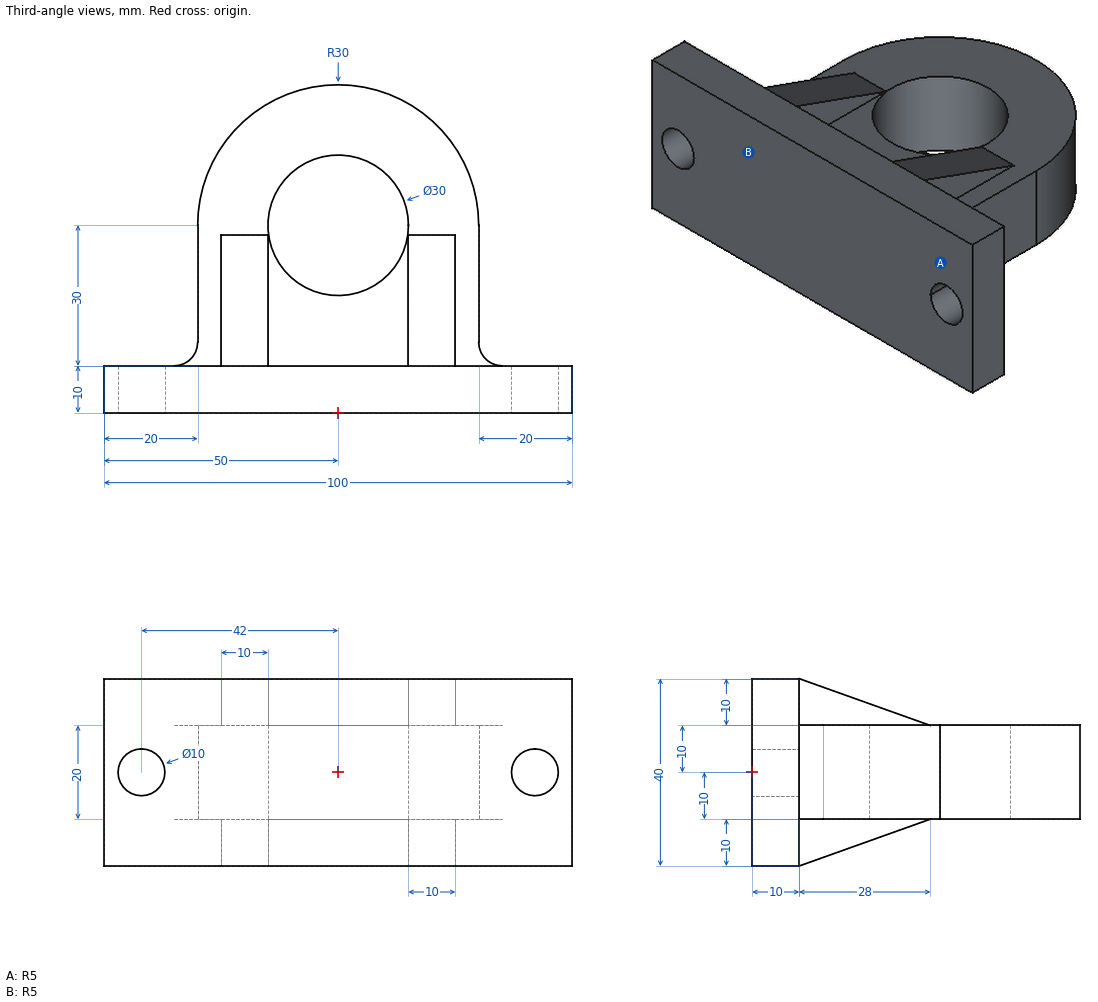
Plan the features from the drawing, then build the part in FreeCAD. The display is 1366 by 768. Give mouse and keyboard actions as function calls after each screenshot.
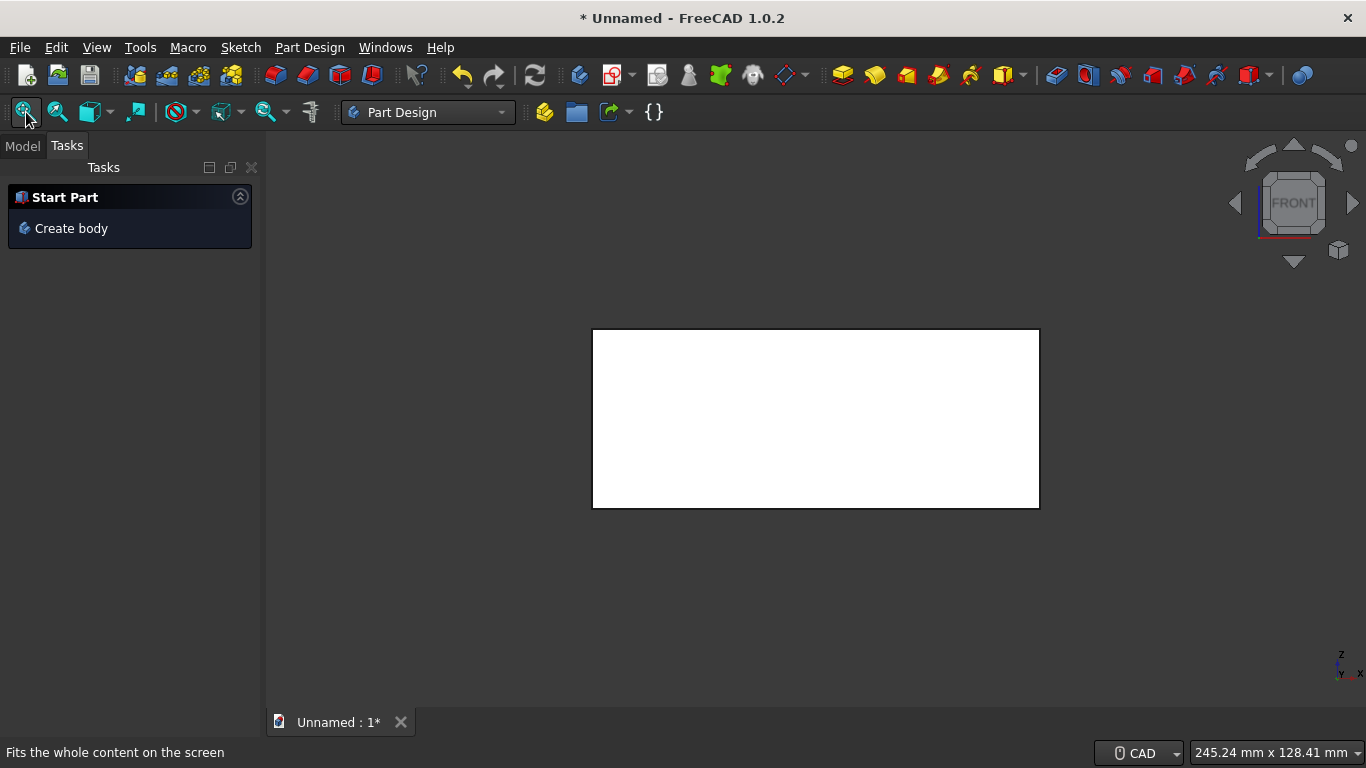
click(26, 112)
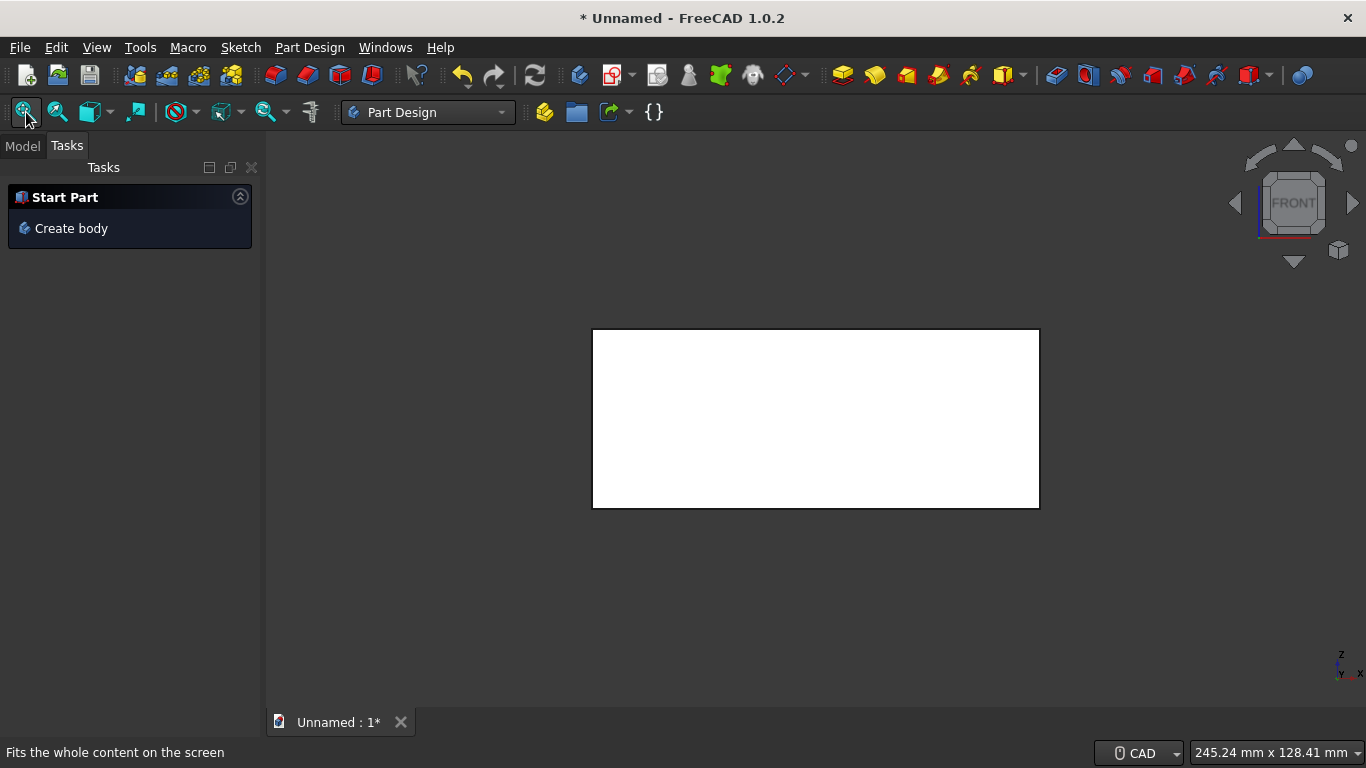
key(3)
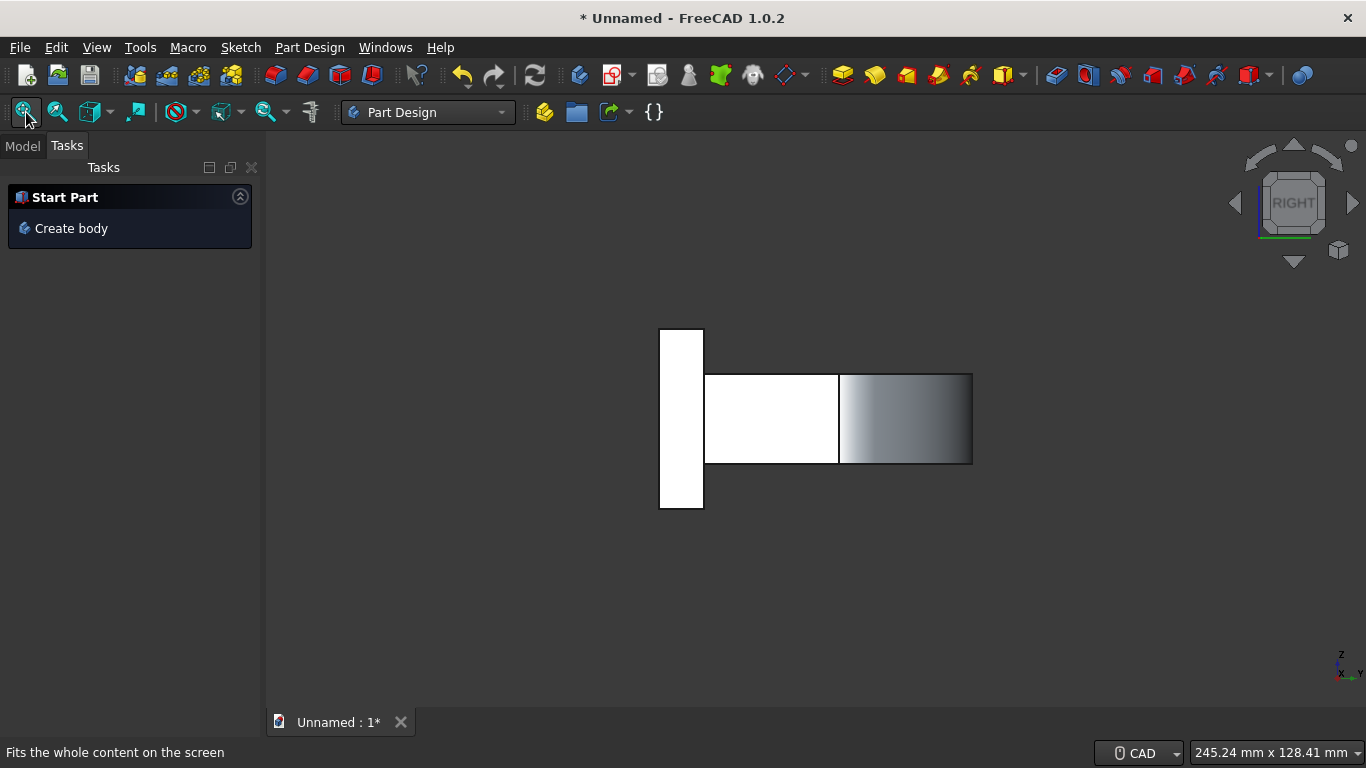
click(26, 112)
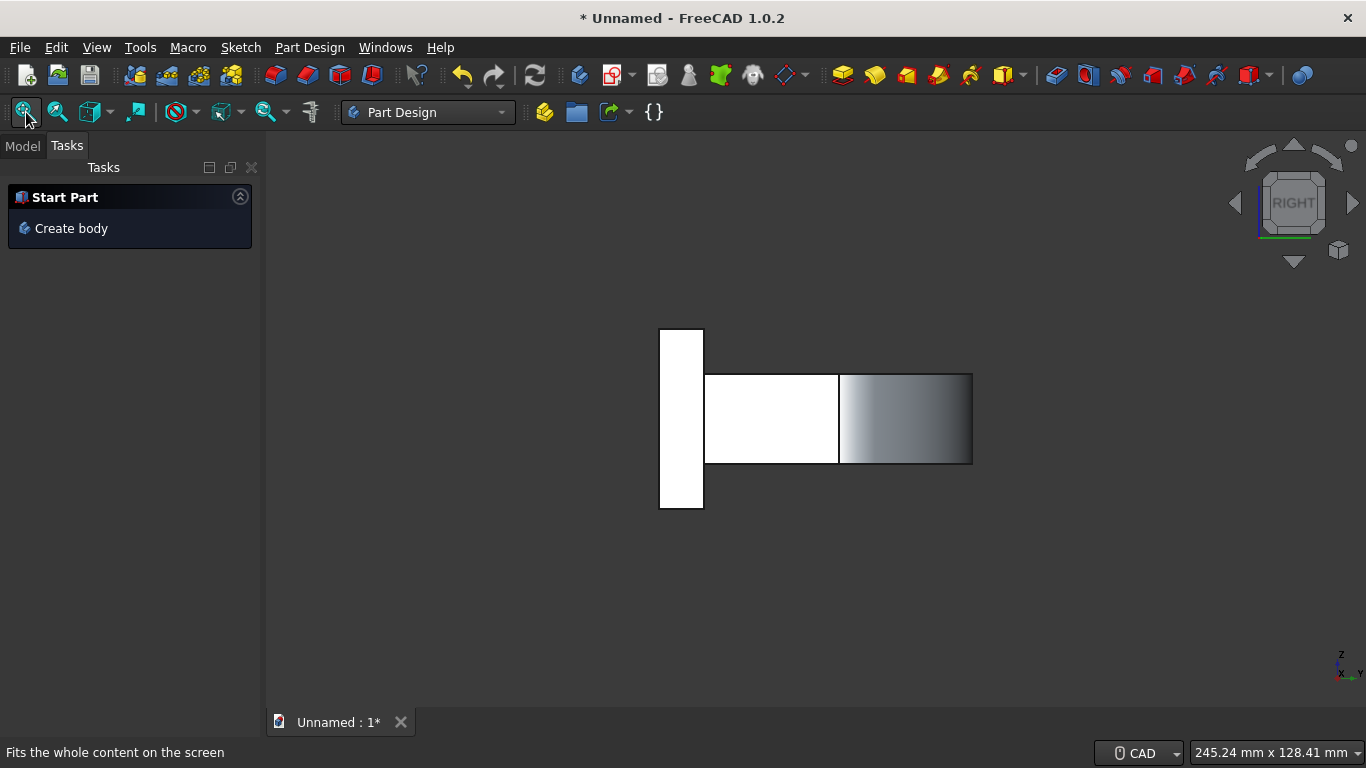
key(5)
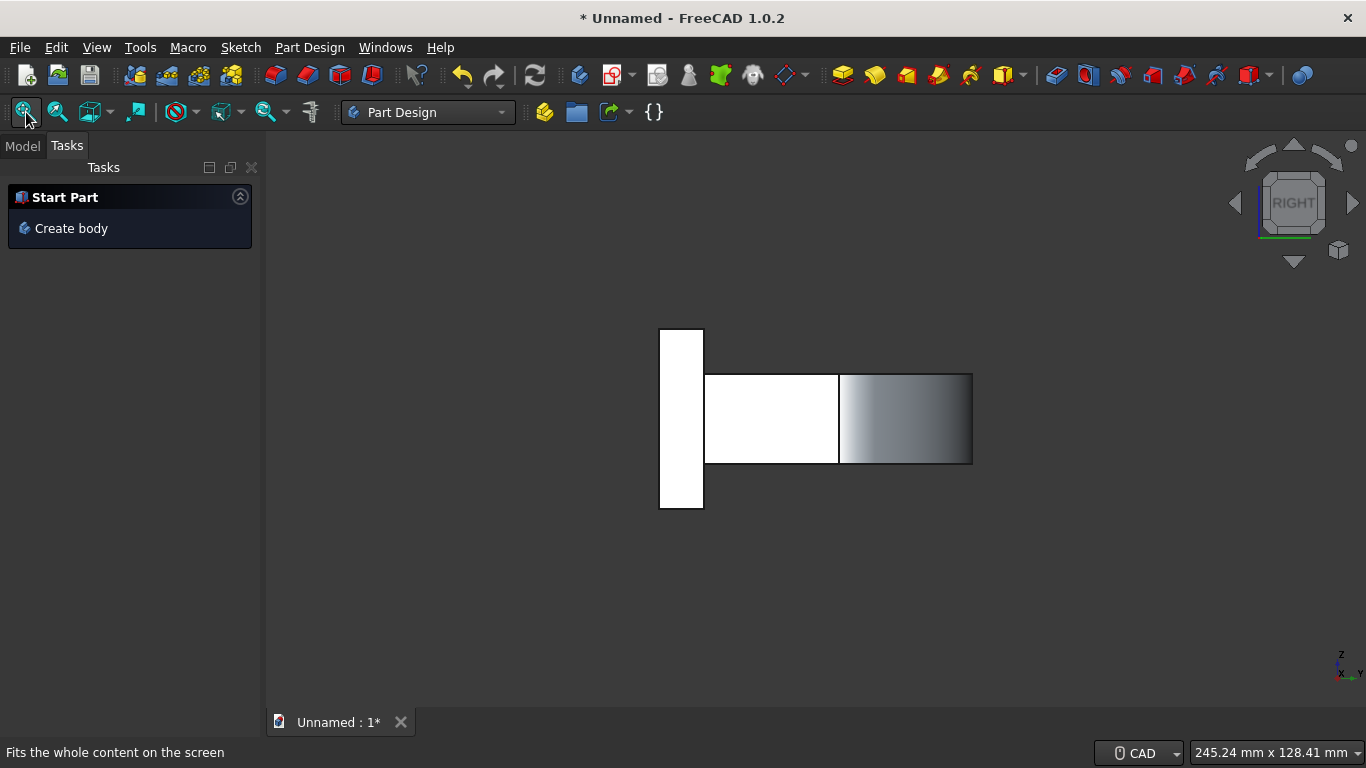
key(4)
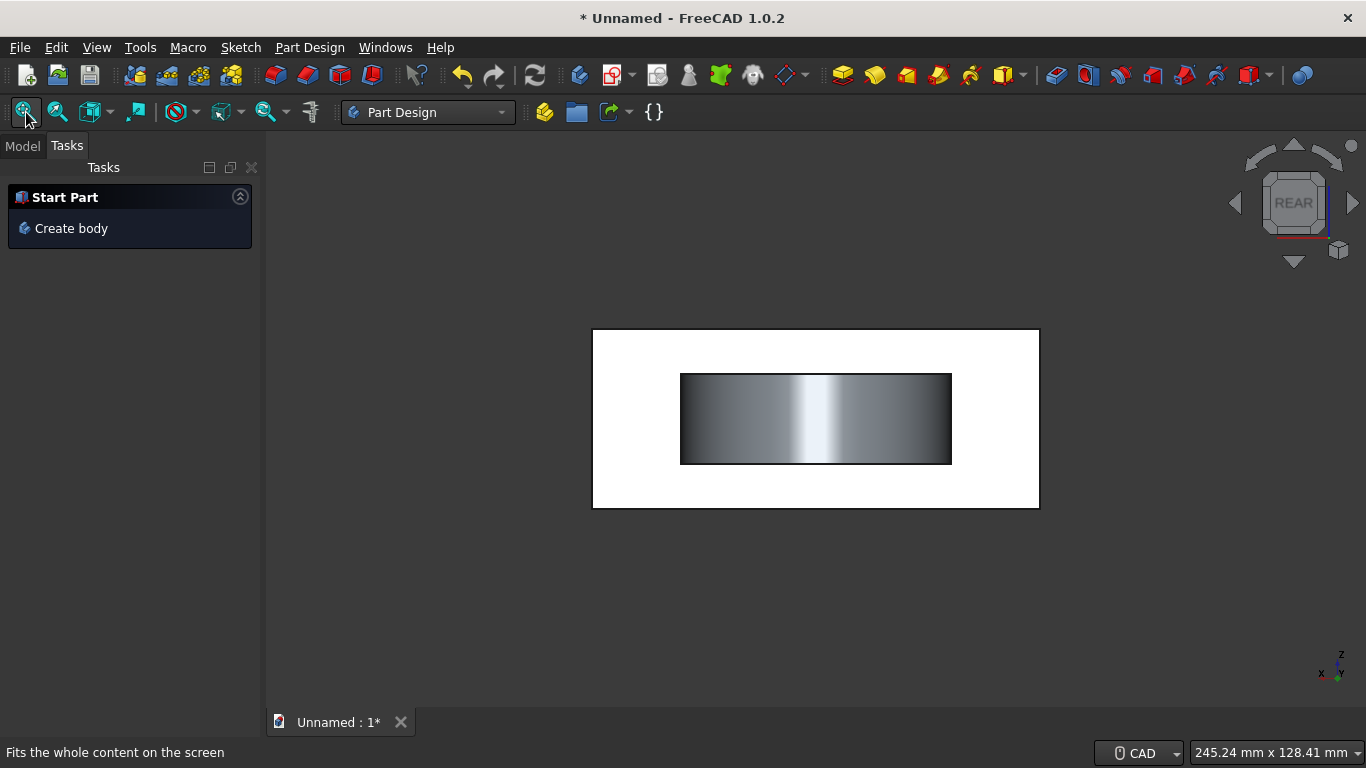
key(v)
key(f)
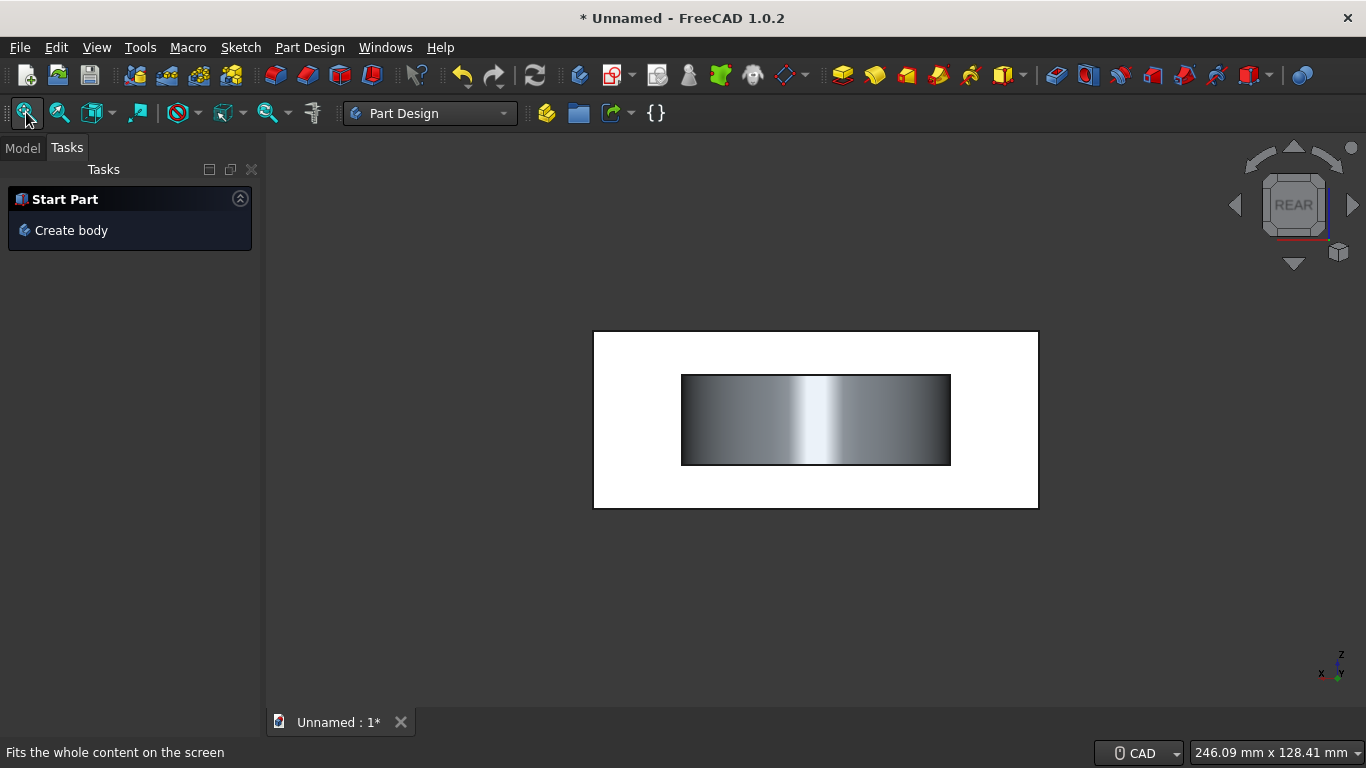
key(6)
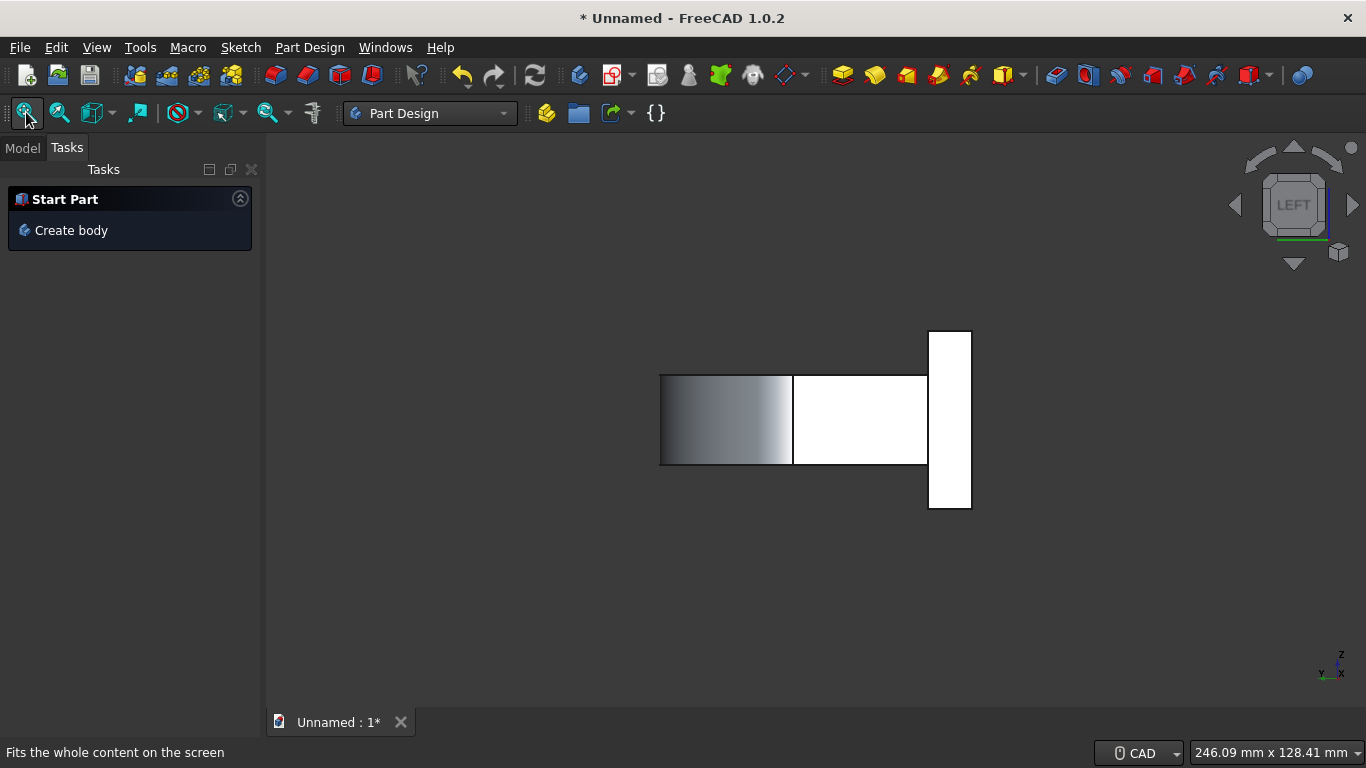
click(28, 114)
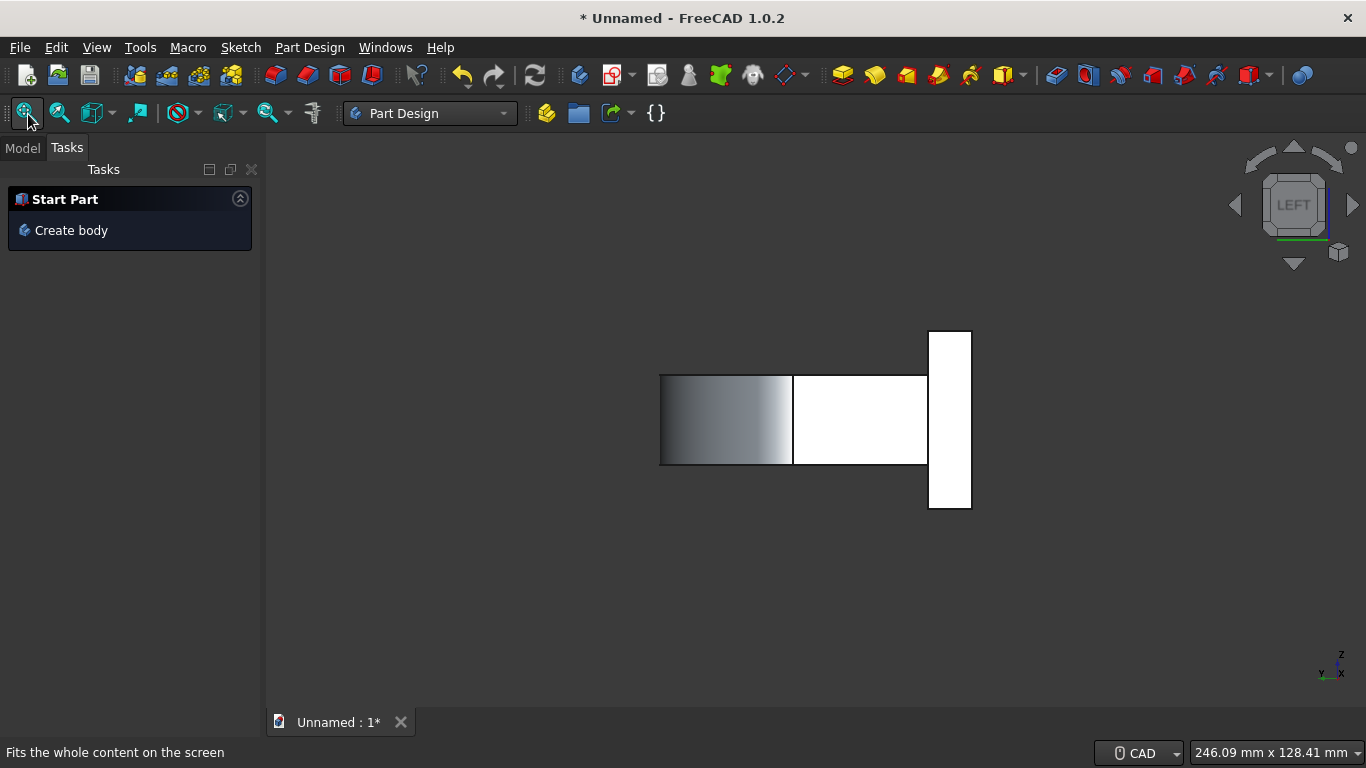
key(v)
key(3)